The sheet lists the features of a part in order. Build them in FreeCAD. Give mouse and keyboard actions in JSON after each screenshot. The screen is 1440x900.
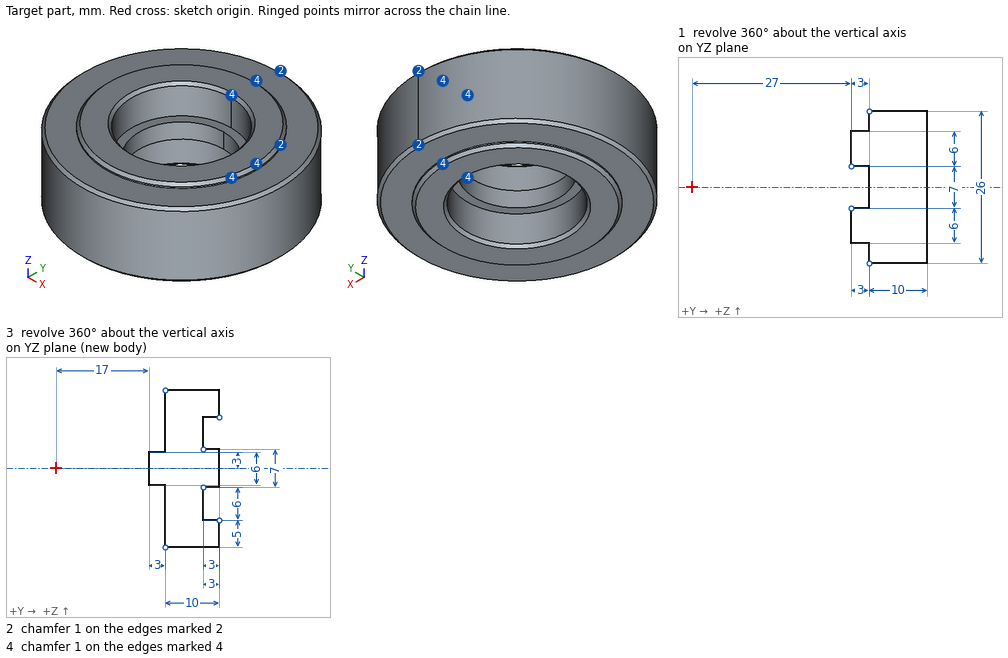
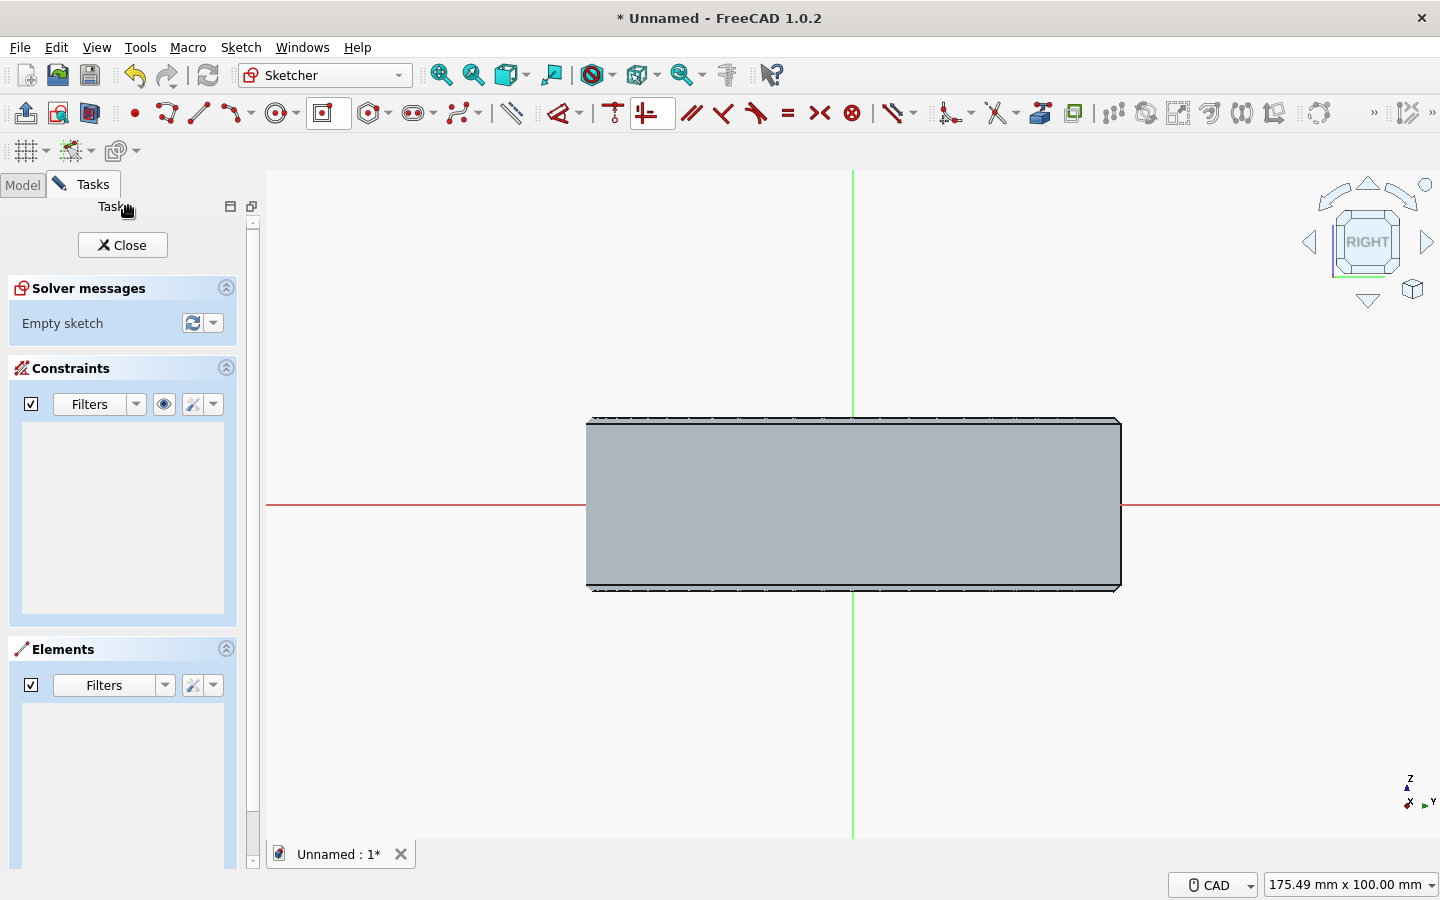
{"action": "scroll", "coordinate": [1091, 504], "scroll_direction": "up", "scroll_amount": 4}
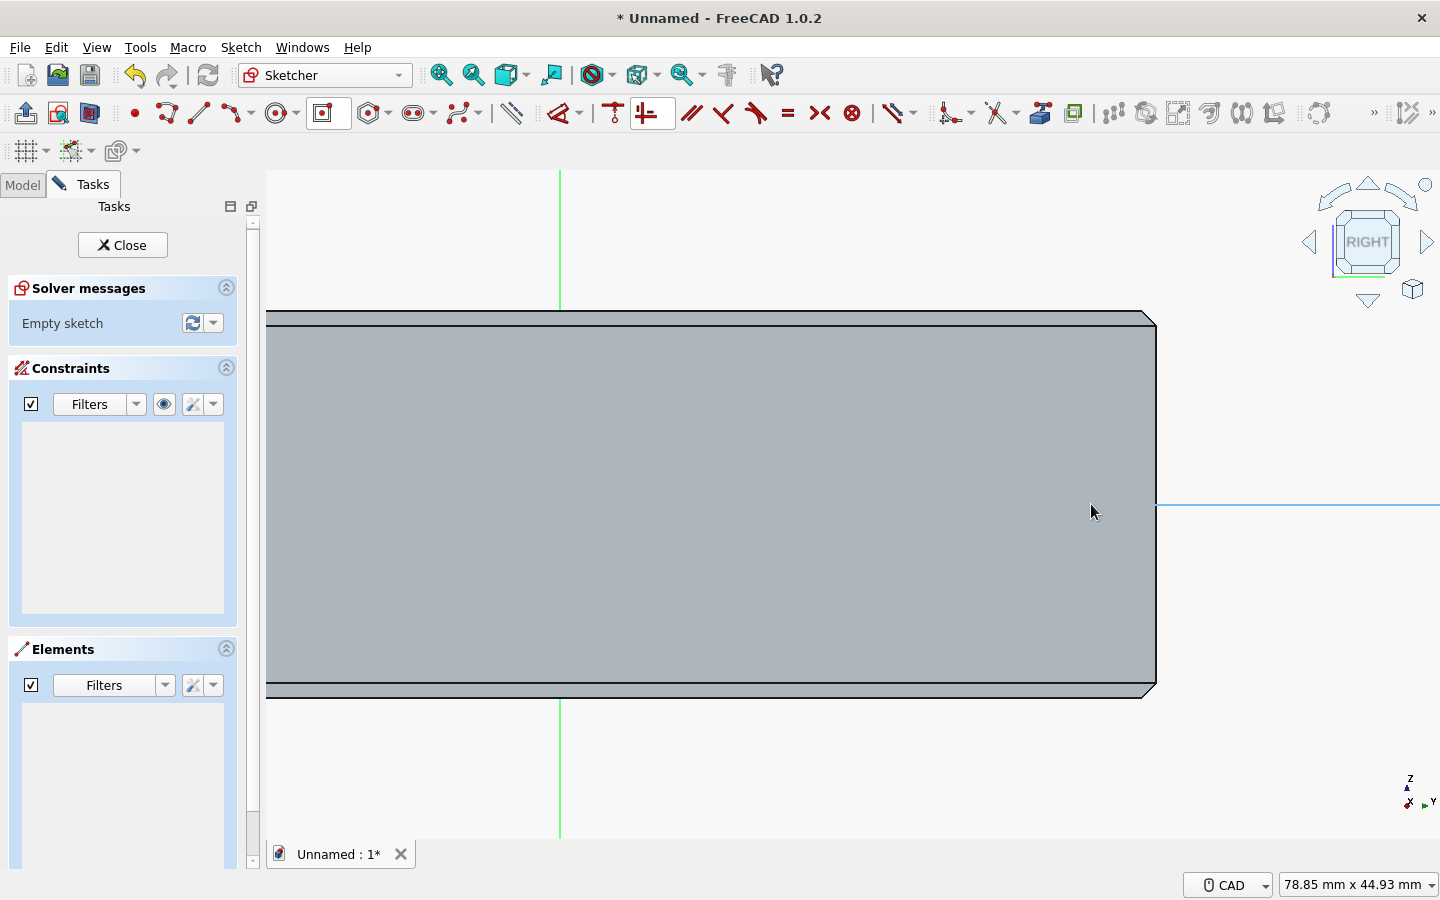
{"action": "left_click", "coordinate": [168, 114]}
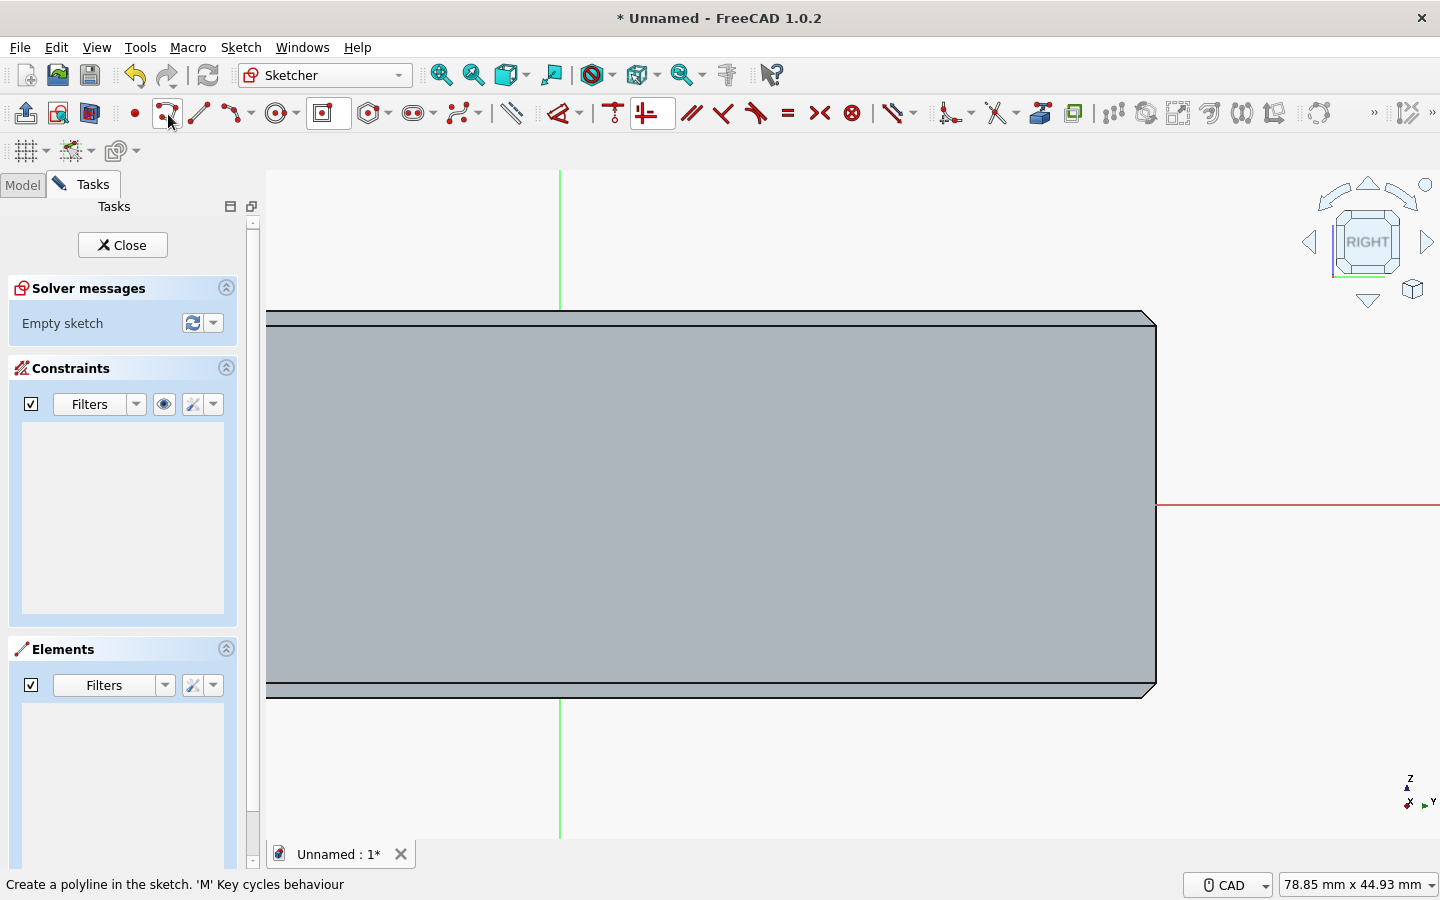
{"action": "left_click", "coordinate": [814, 460]}
{"action": "left_click", "coordinate": [814, 549]}
{"action": "left_click", "coordinate": [858, 549]}
{"action": "left_click", "coordinate": [858, 720]}
{"action": "left_click", "coordinate": [1007, 720]}
{"action": "left_click", "coordinate": [1007, 646]}
{"action": "left_click", "coordinate": [962, 646]}
{"action": "left_click", "coordinate": [962, 557]}
{"action": "left_click", "coordinate": [1007, 557]}
{"action": "left_click", "coordinate": [1007, 452]}
{"action": "left_click", "coordinate": [962, 452]}
{"action": "left_click", "coordinate": [962, 363]}
{"action": "left_click", "coordinate": [1007, 363]}
{"action": "left_click", "coordinate": [1007, 289]}
{"action": "left_click", "coordinate": [858, 289]}
{"action": "left_click", "coordinate": [858, 460]}
{"action": "left_click", "coordinate": [814, 461]}
{"action": "key", "text": "Escape"}
{"action": "key", "text": "Escape"}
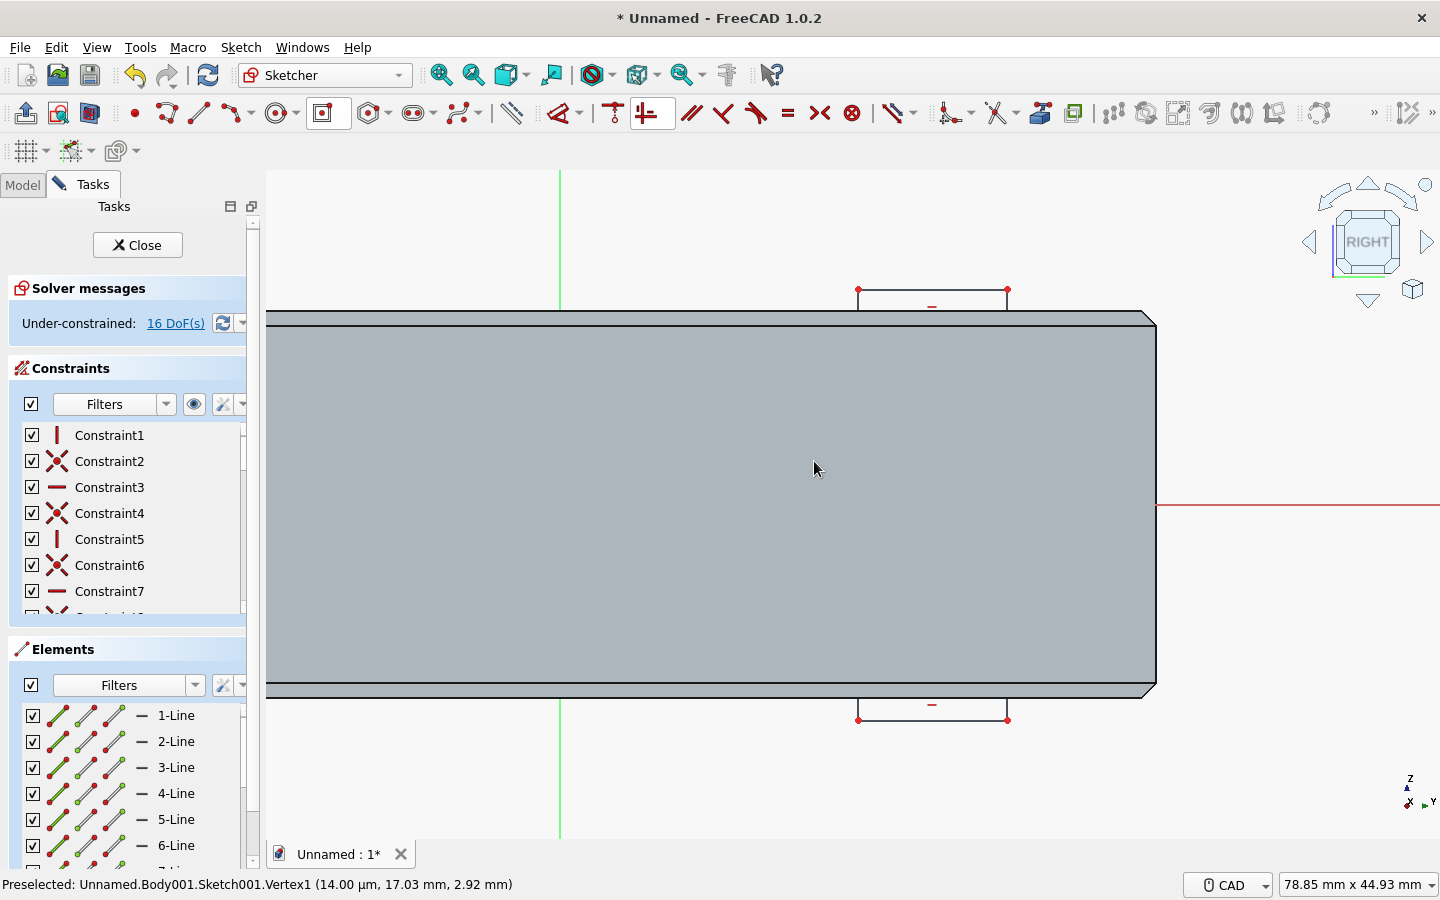
{"action": "left_click", "coordinate": [962, 558]}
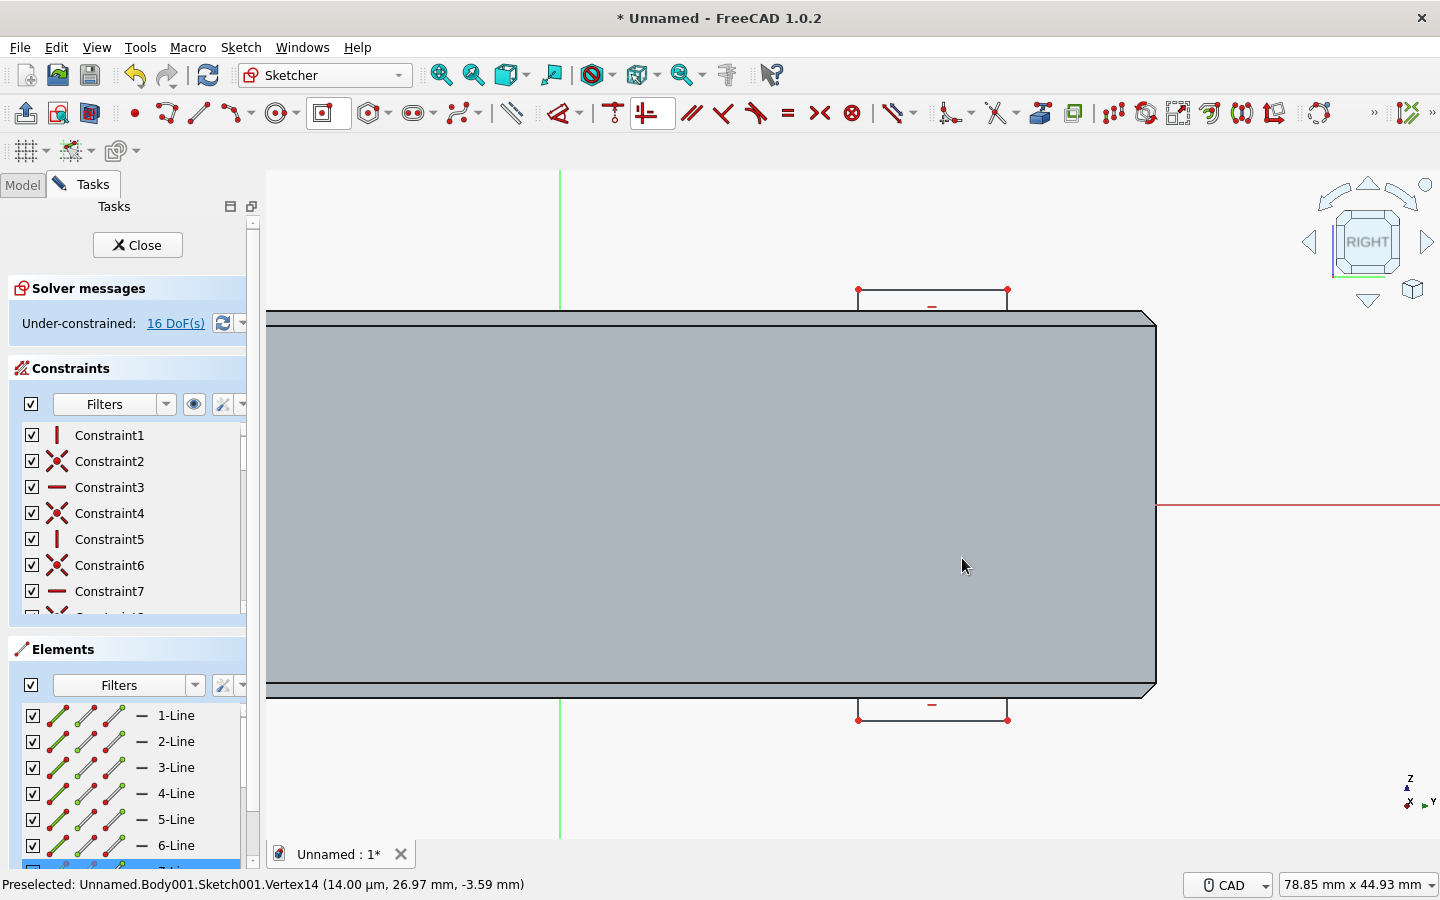
{"action": "left_click", "coordinate": [962, 453]}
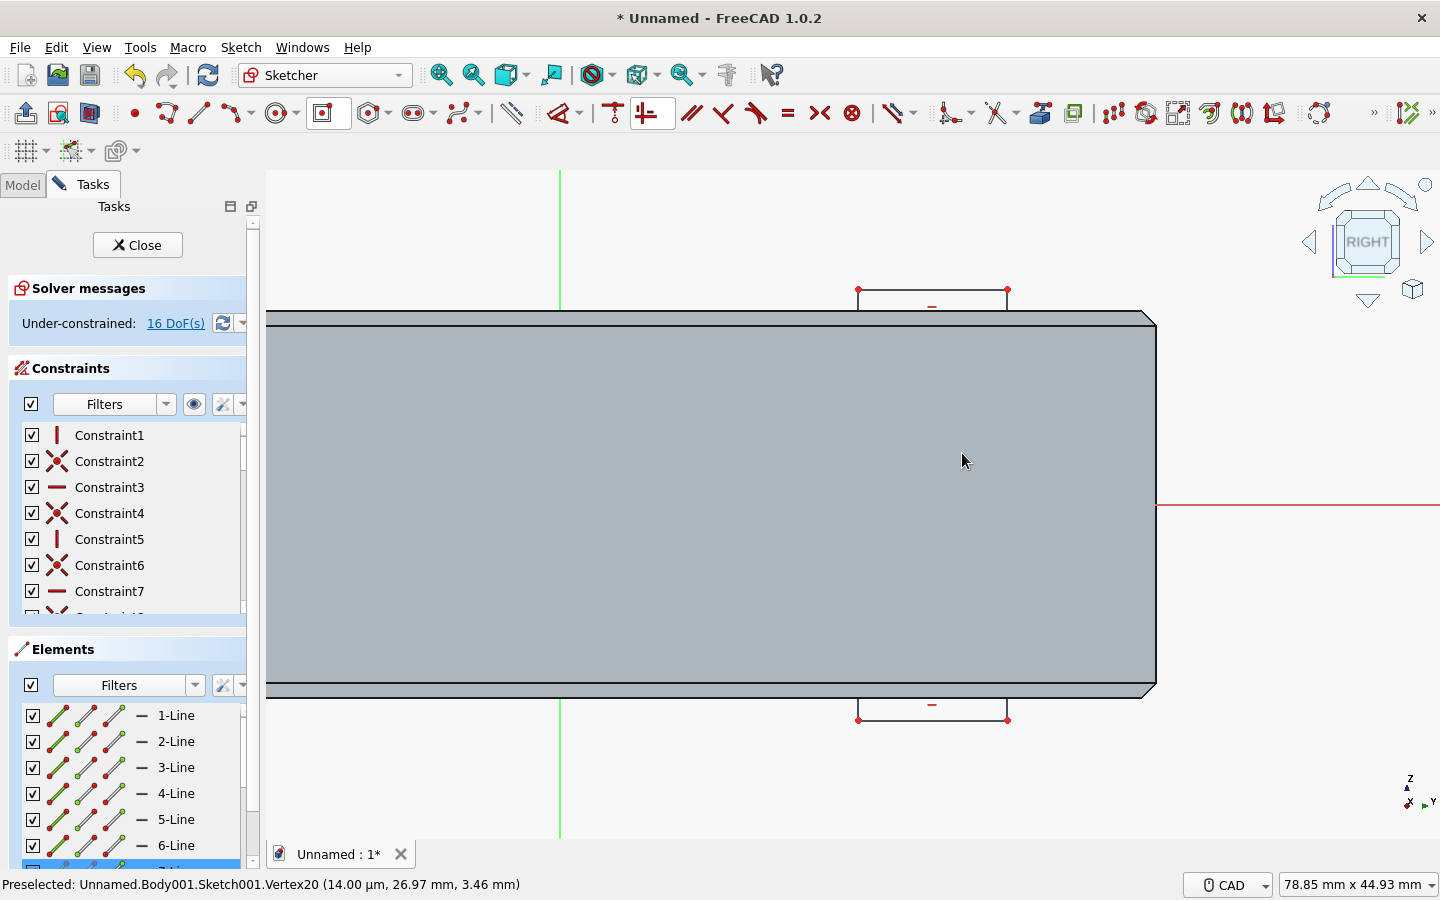
{"action": "left_click", "coordinate": [364, 504]}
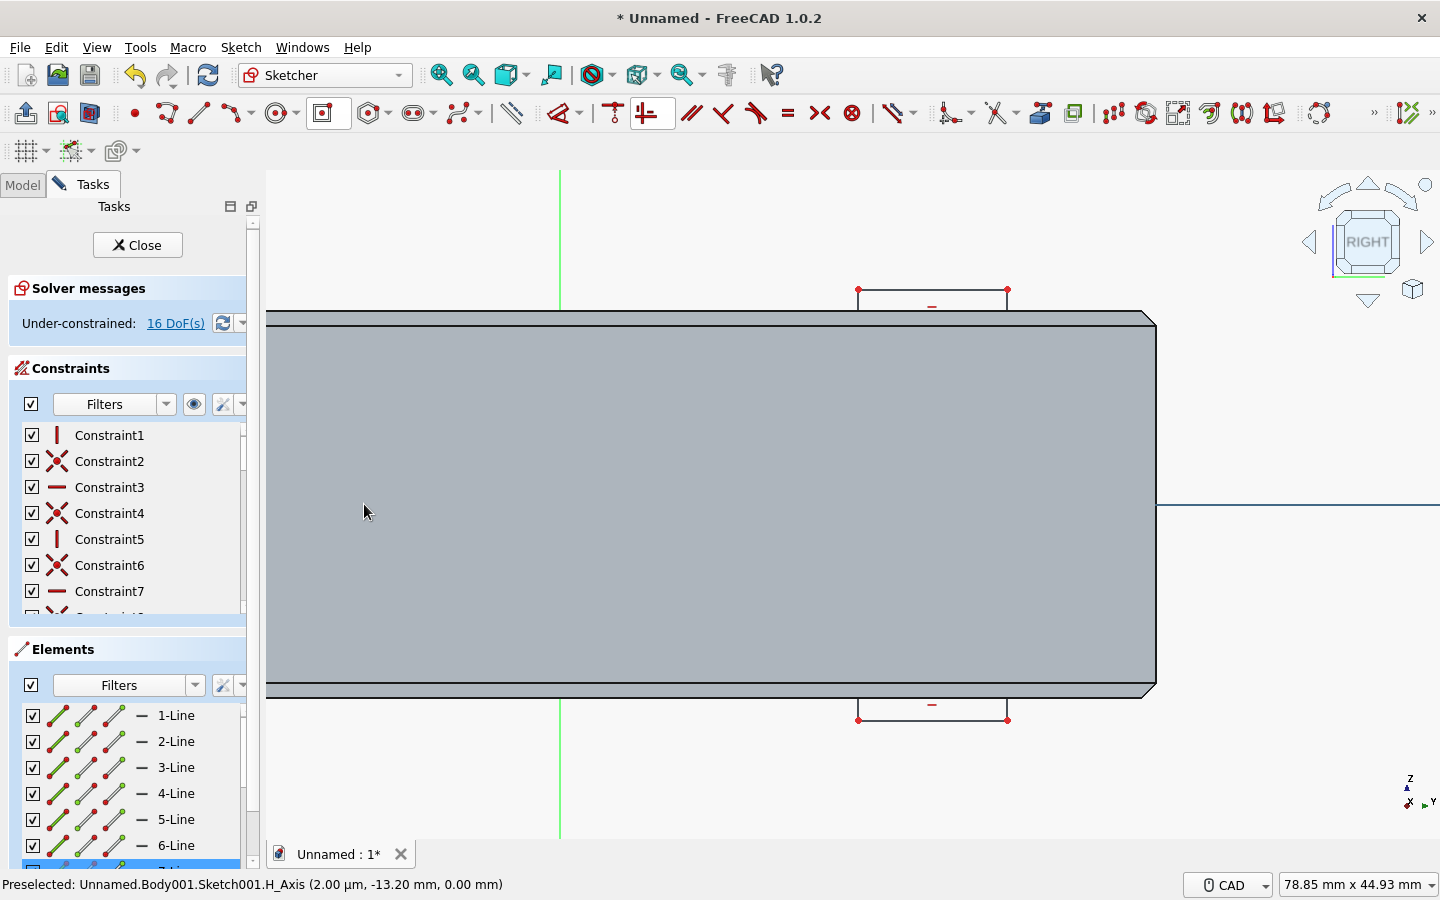
{"action": "left_click", "coordinate": [820, 114]}